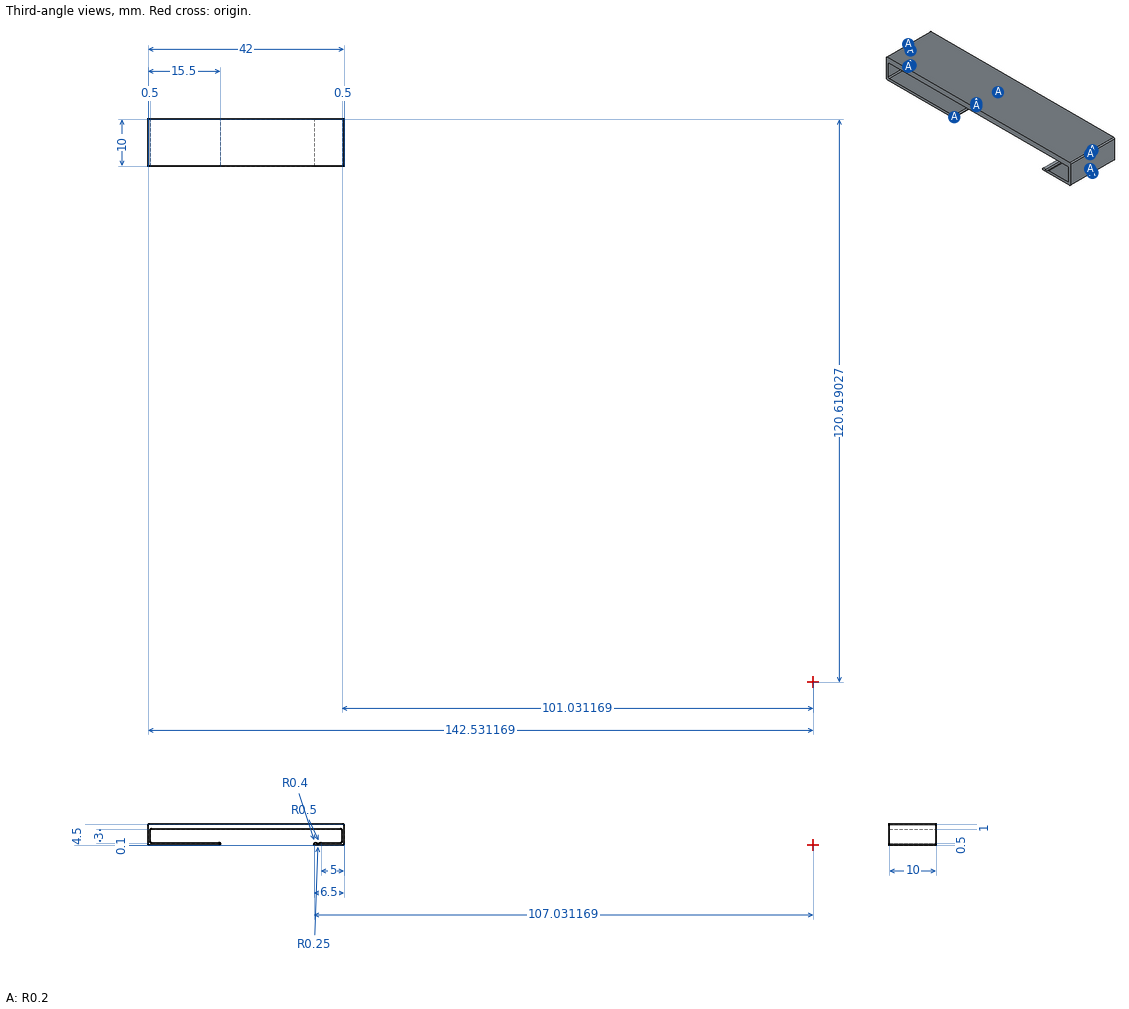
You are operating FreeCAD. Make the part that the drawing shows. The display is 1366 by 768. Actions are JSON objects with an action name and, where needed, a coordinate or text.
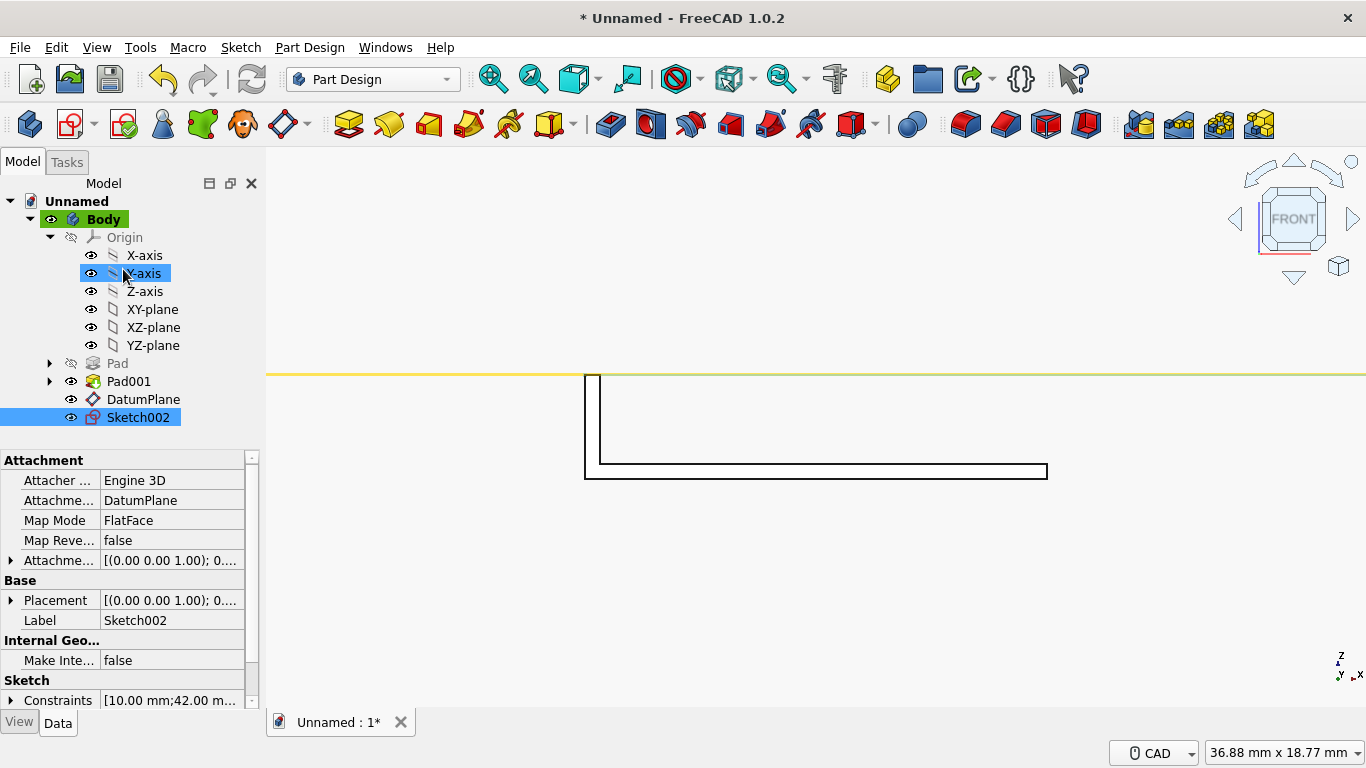
{"action": "left_click", "coordinate": [350, 124]}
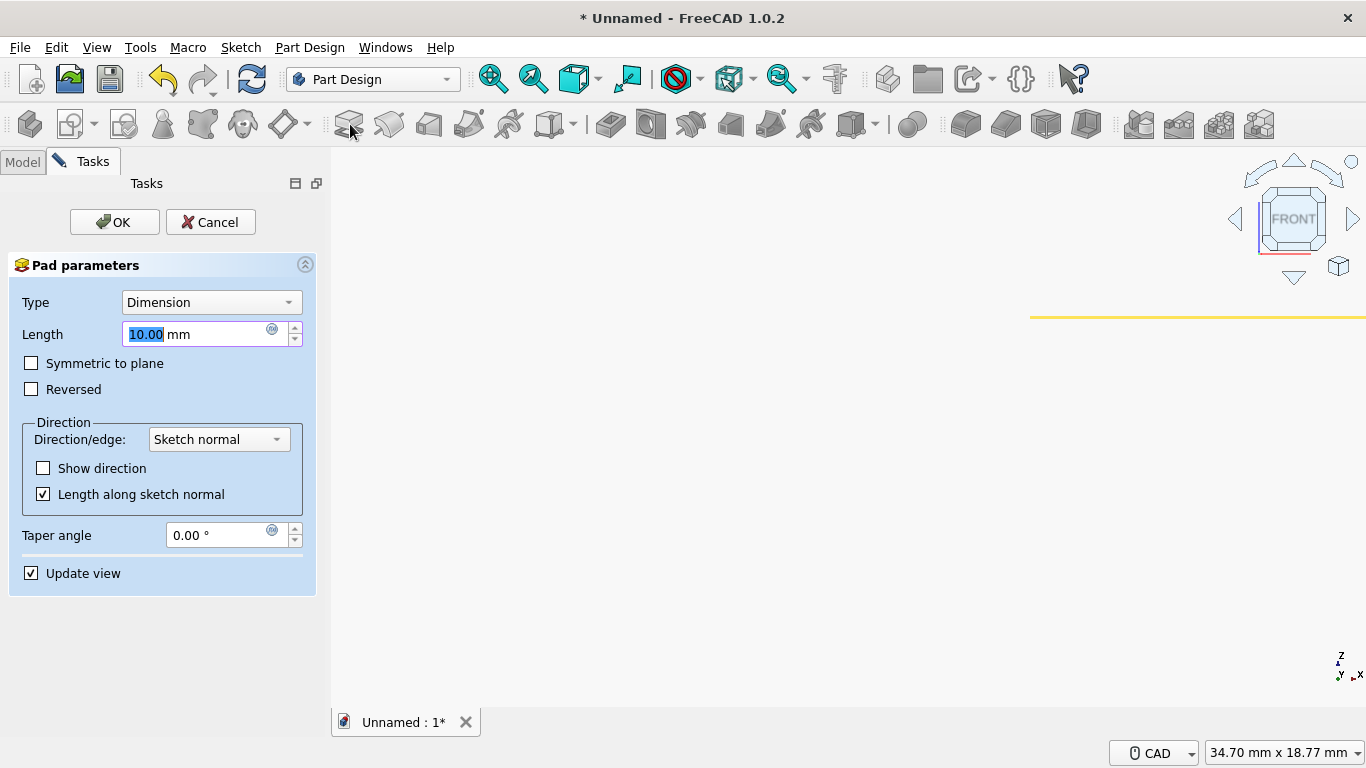
{"action": "type", "text": "1"}
{"action": "key", "text": "Tab"}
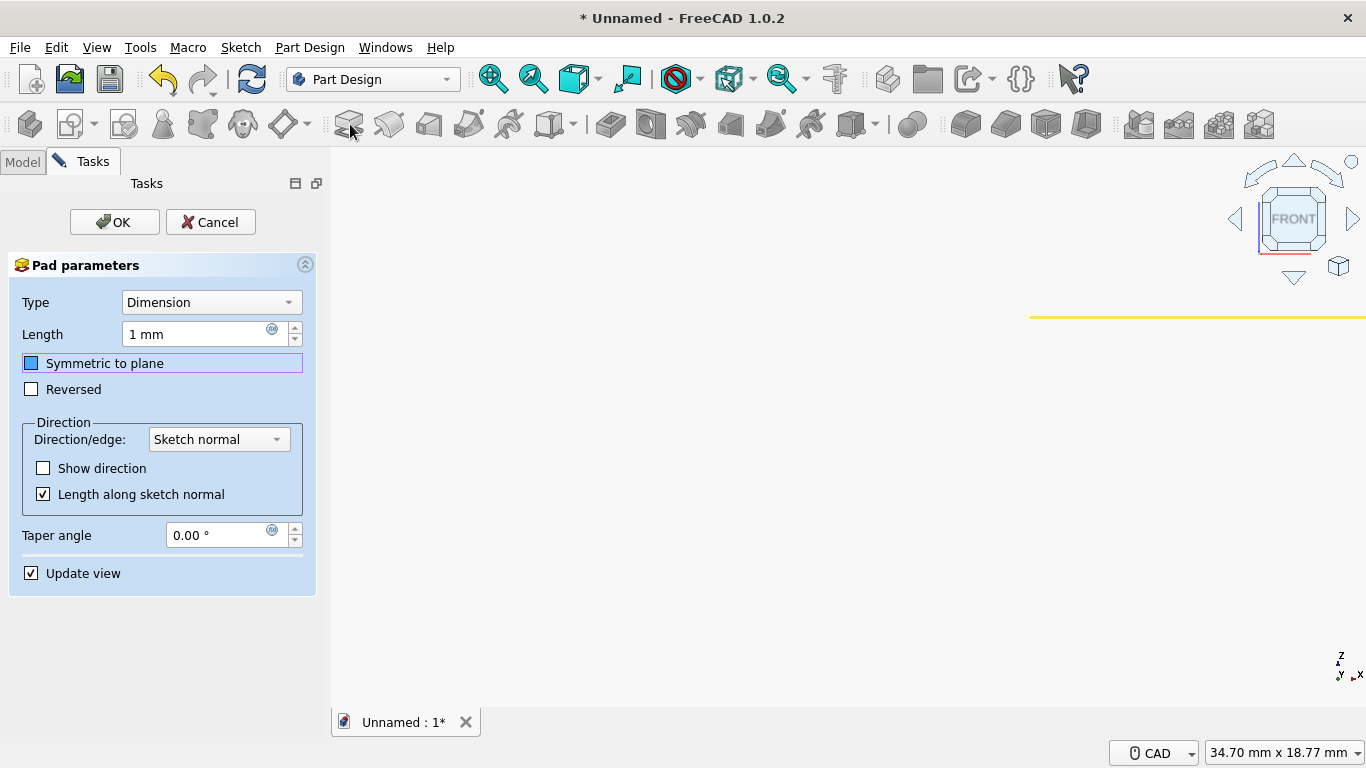
{"action": "left_click", "coordinate": [115, 222]}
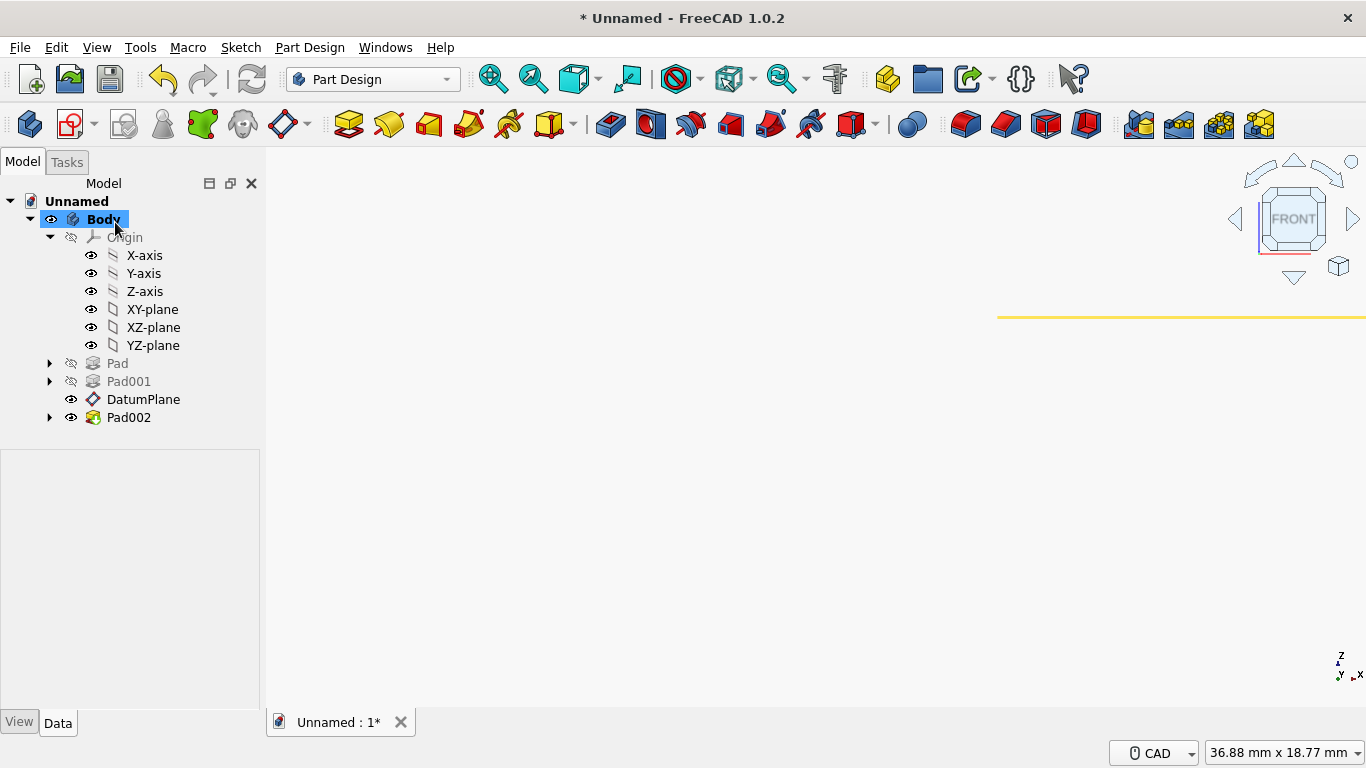
{"action": "left_click", "coordinate": [116, 399]}
{"action": "key", "text": "space"}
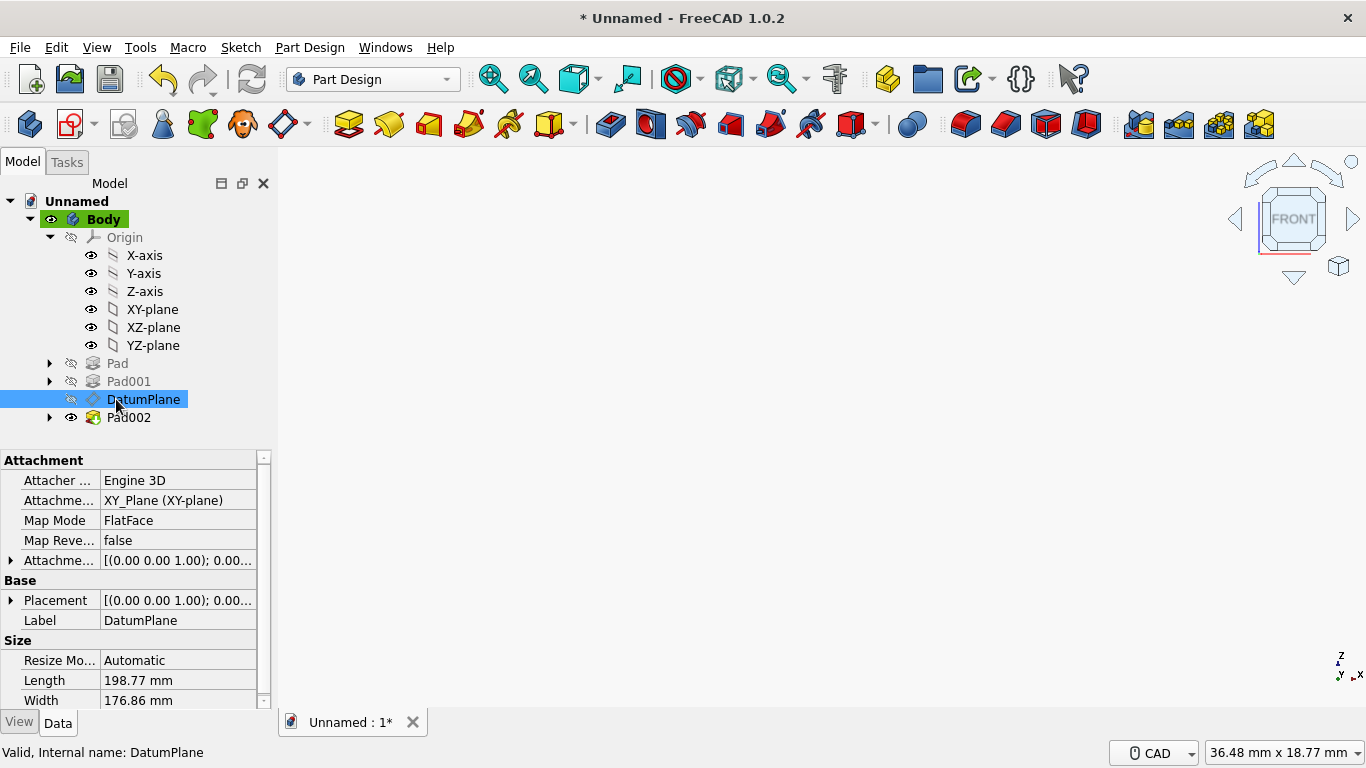
{"action": "left_click", "coordinate": [494, 80]}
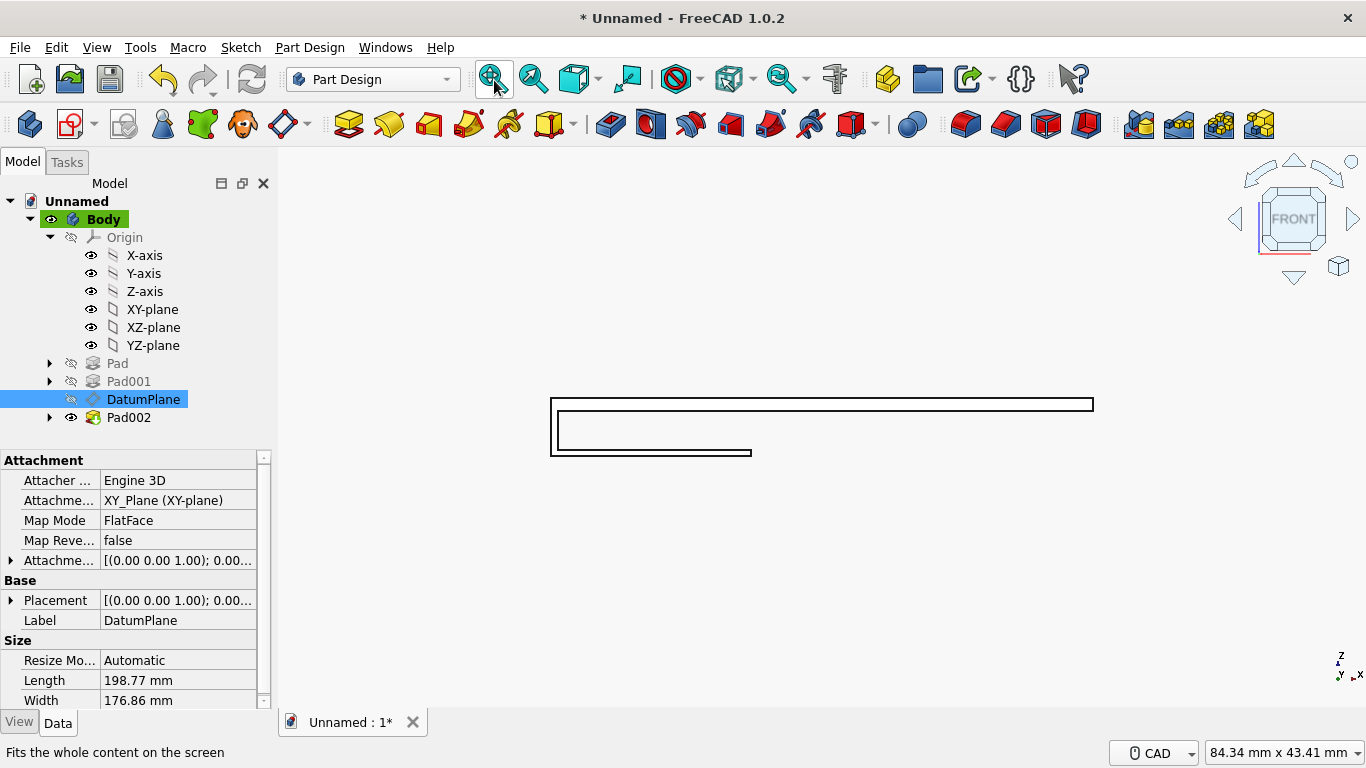
{"action": "key", "text": "0"}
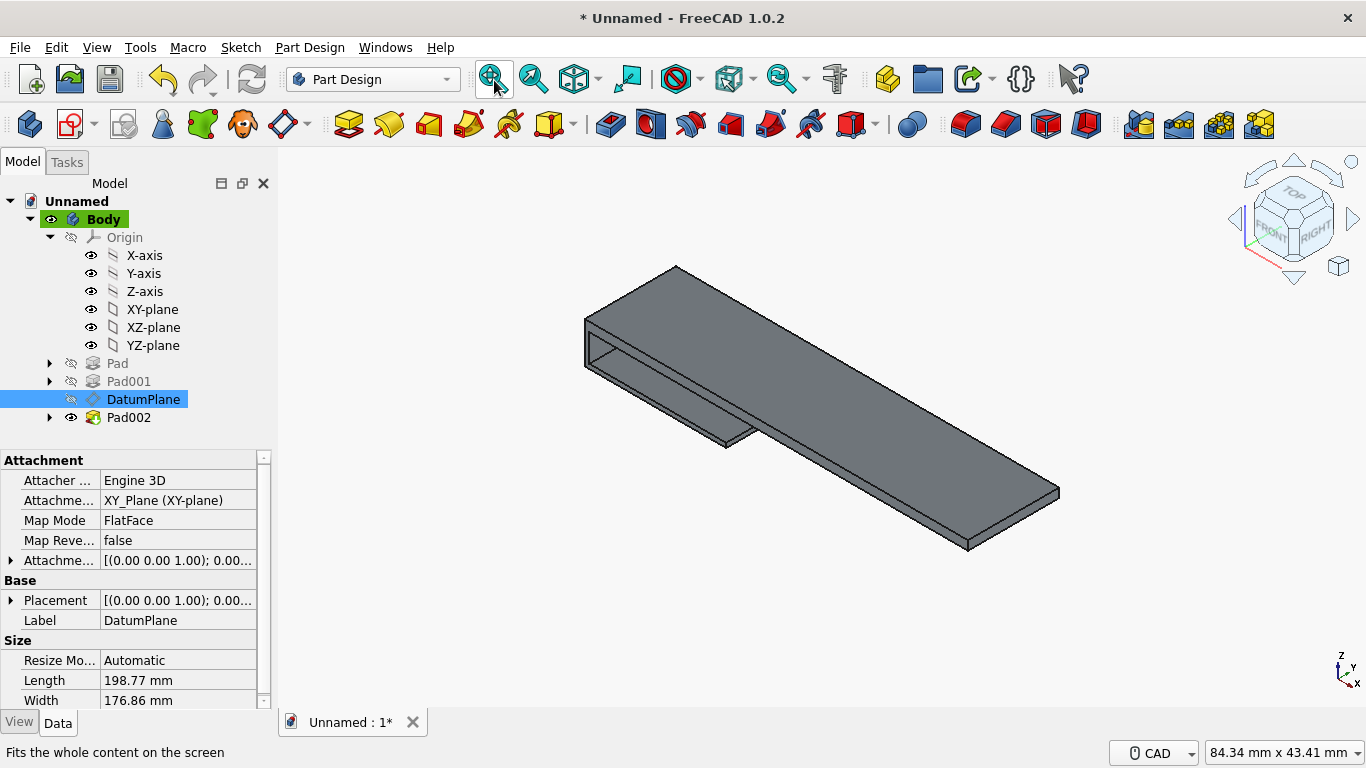
{"action": "left_click", "coordinate": [931, 466]}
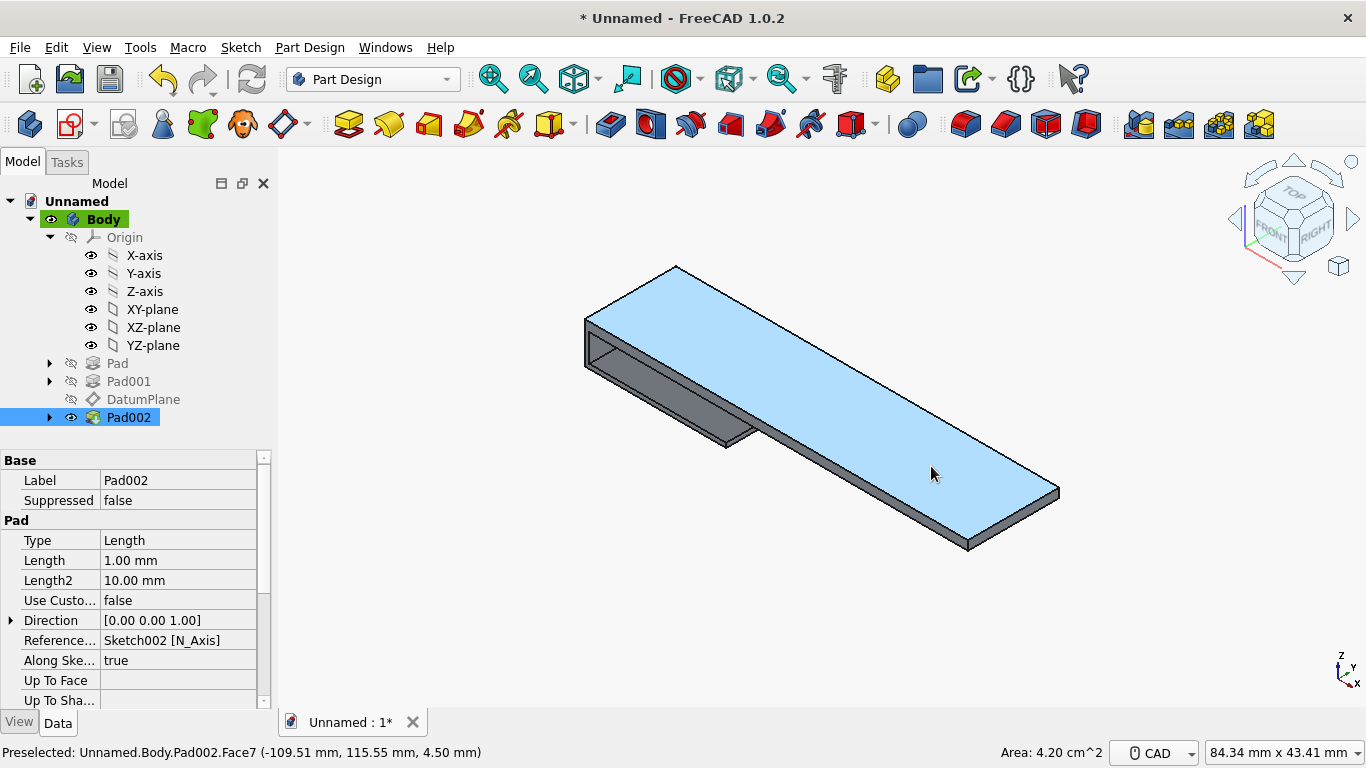
{"action": "left_click", "coordinate": [70, 124]}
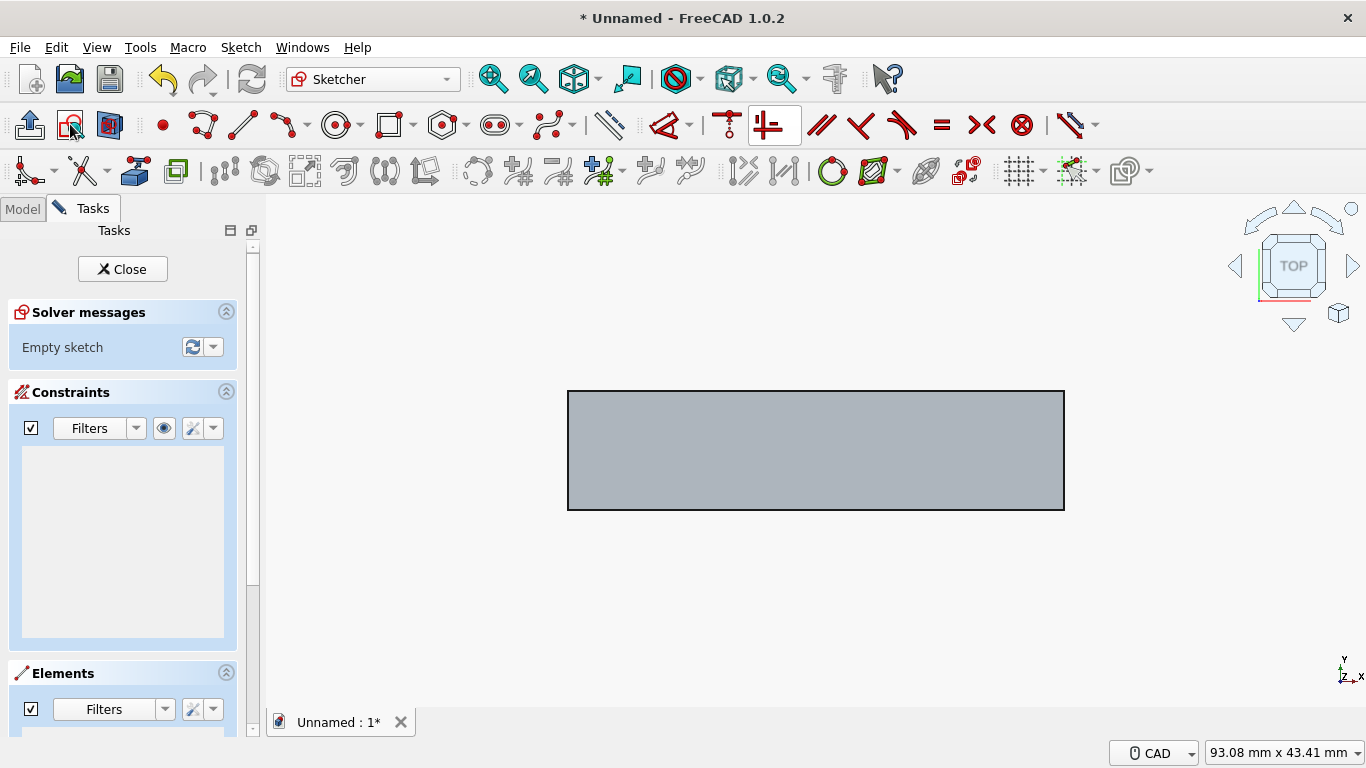
{"action": "scroll", "coordinate": [1201, 451], "scroll_direction": "up", "scroll_amount": 5}